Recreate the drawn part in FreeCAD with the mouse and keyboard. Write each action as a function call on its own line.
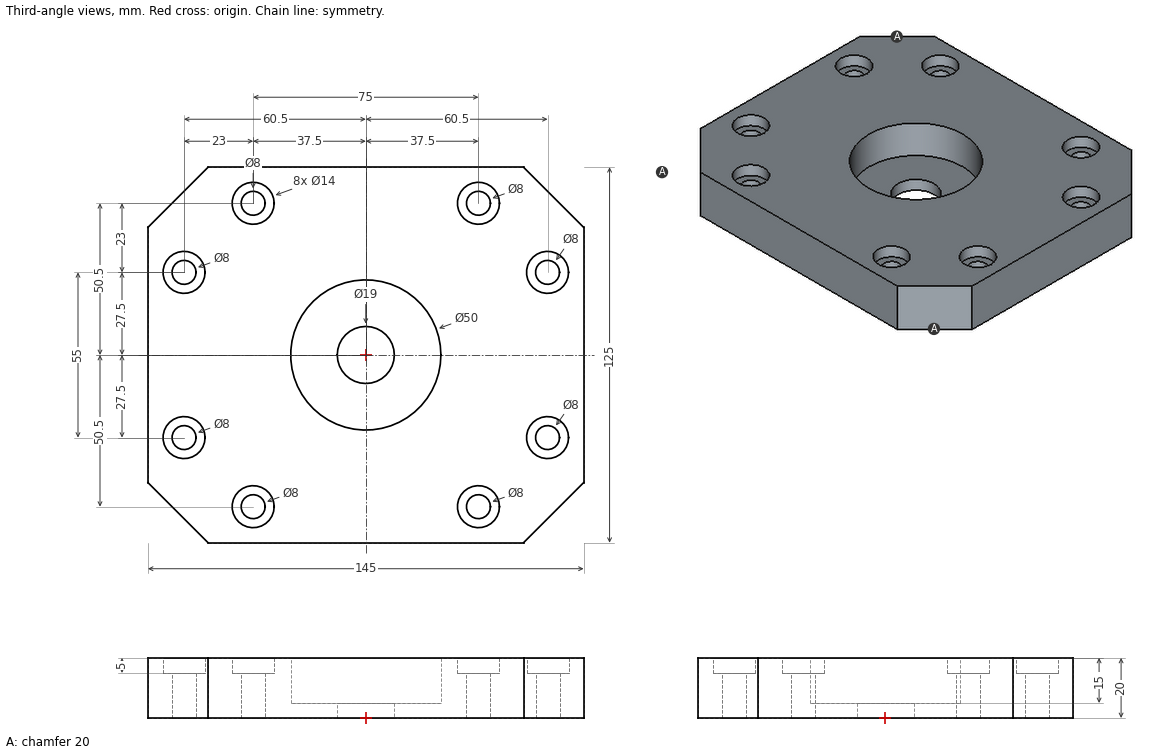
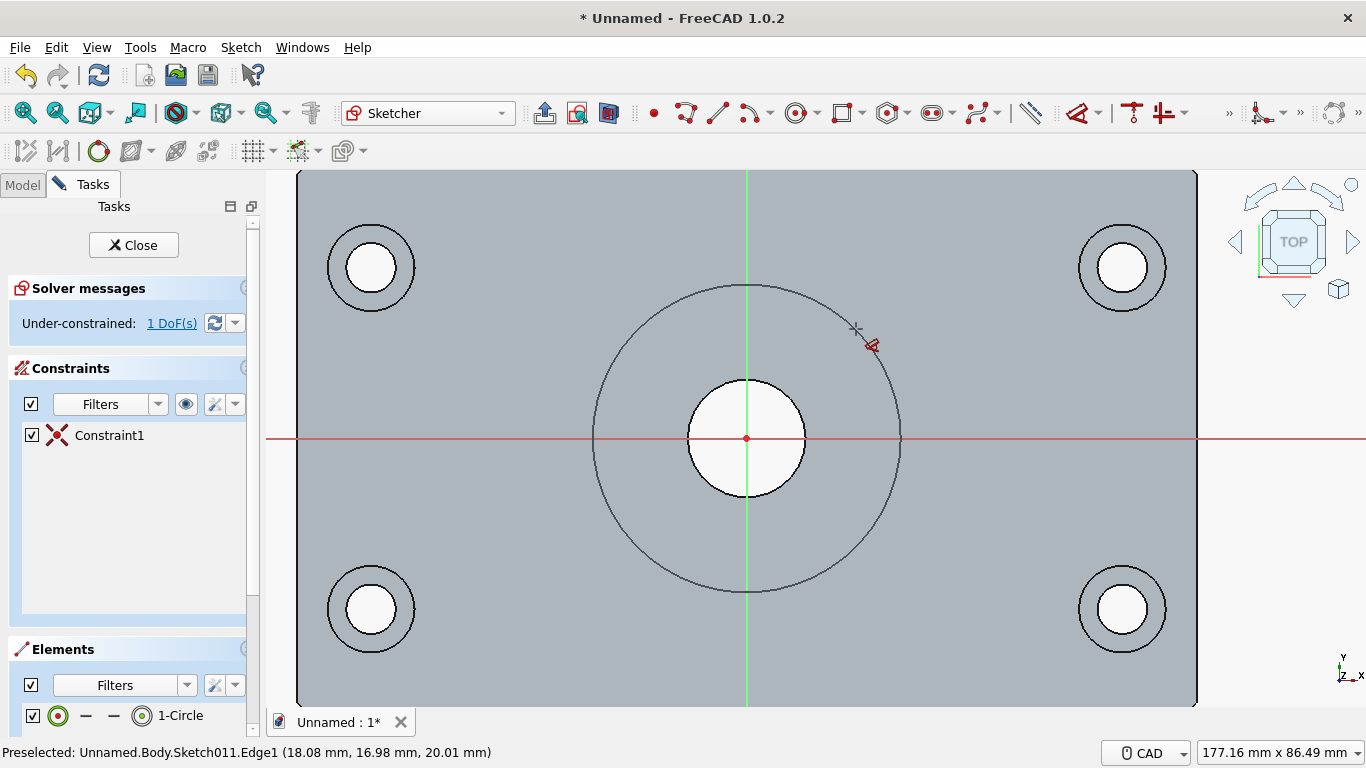
click(855, 329)
click(878, 306)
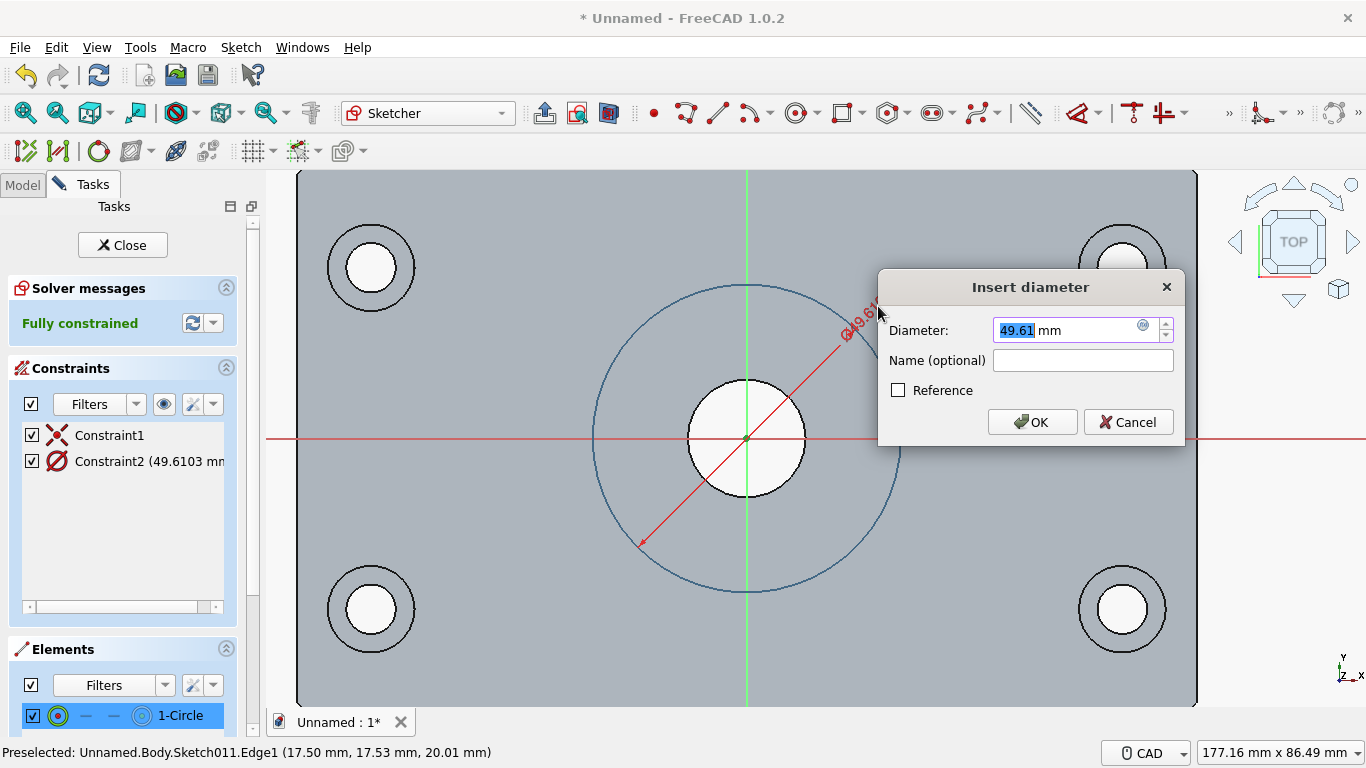
text(50)
key(Return)
key(Escape)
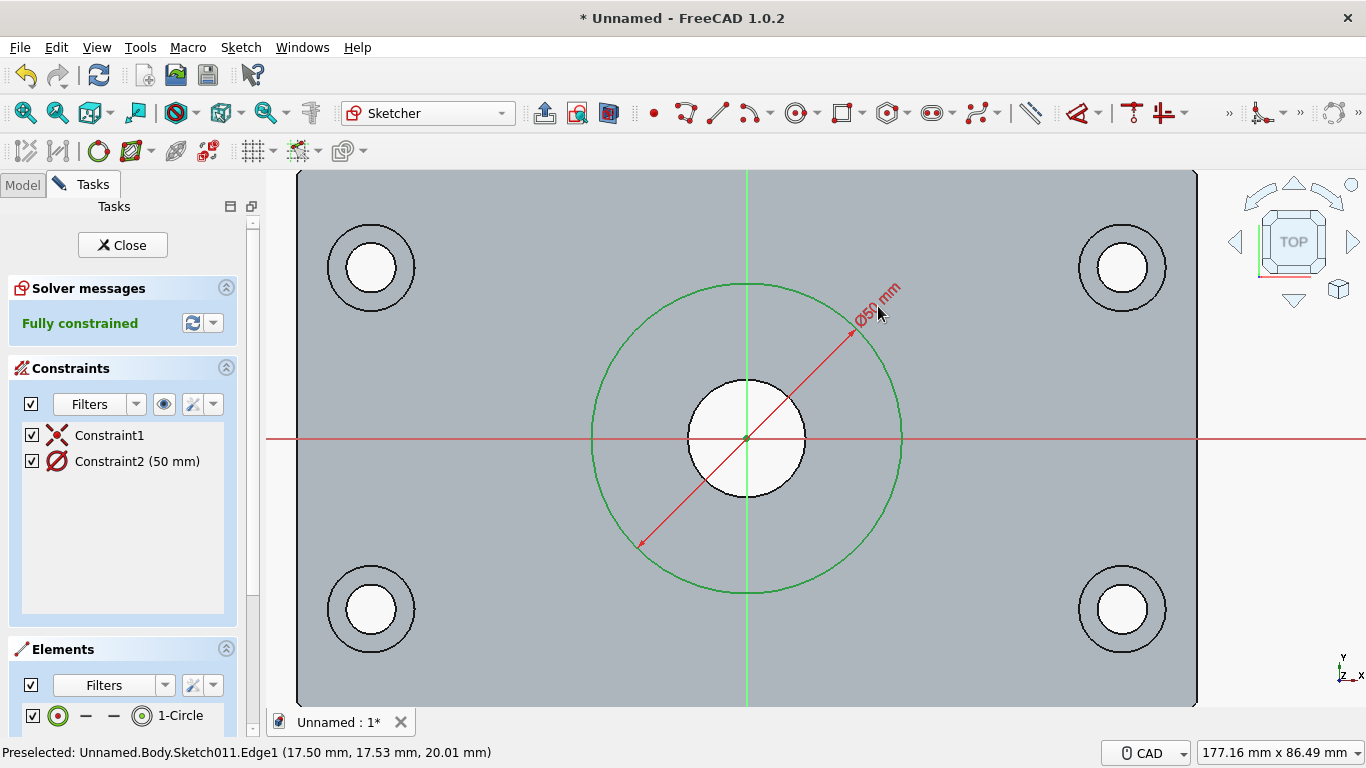
click(123, 245)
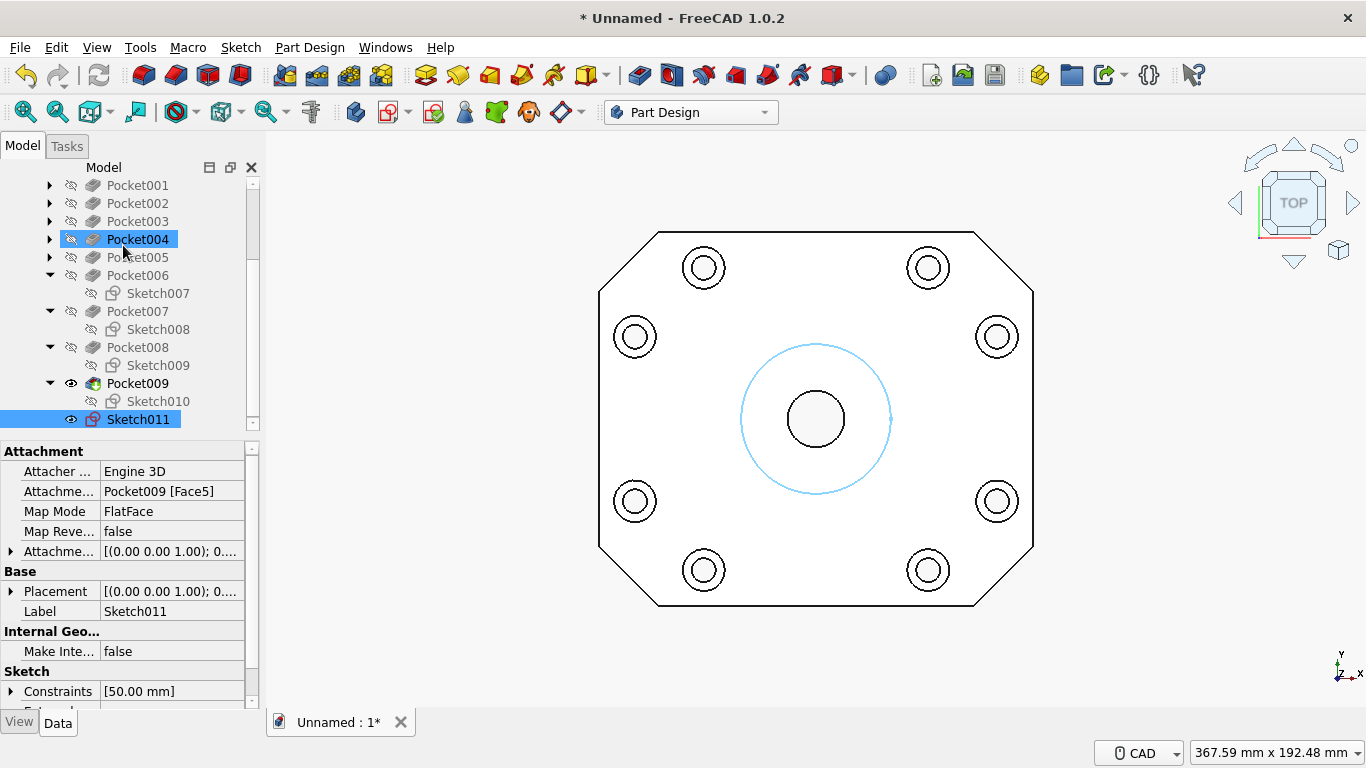
click(640, 76)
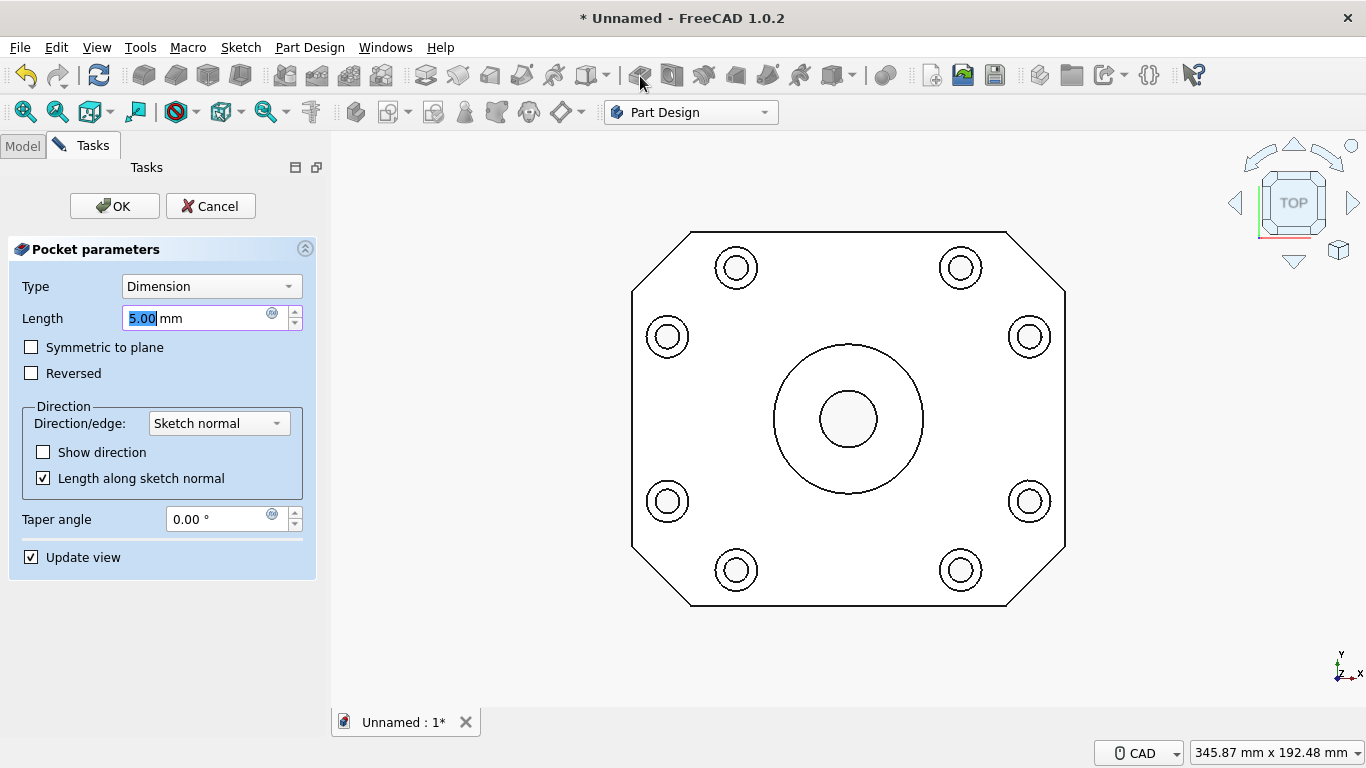
text(15)
key(Tab)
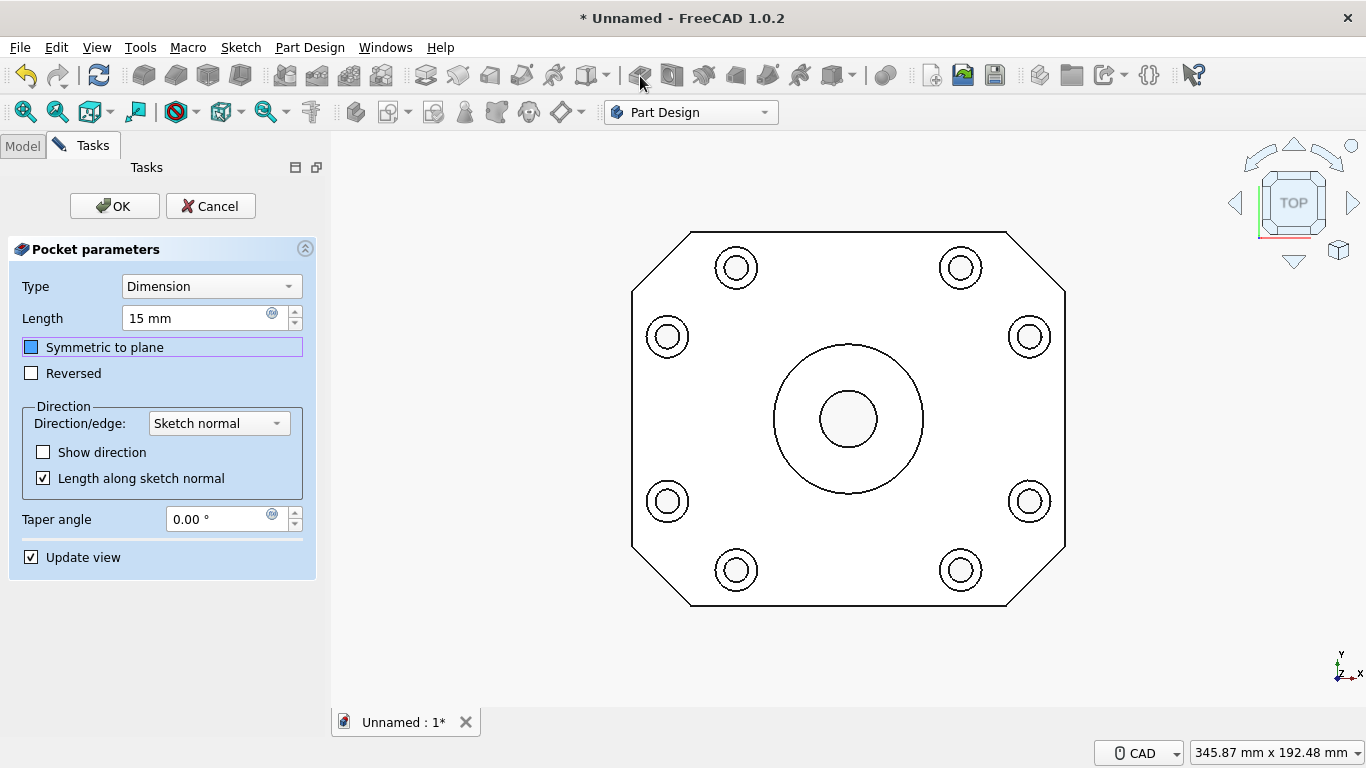
click(115, 206)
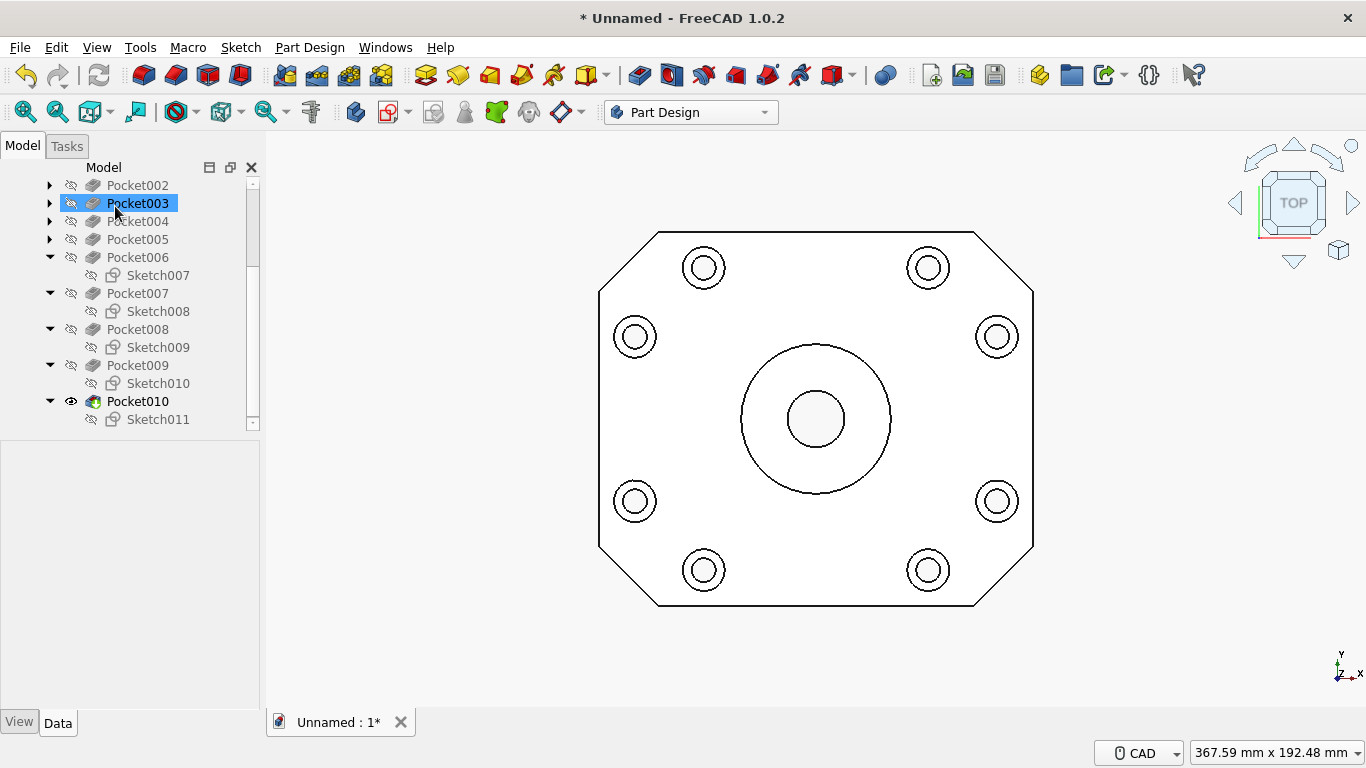
key(0)